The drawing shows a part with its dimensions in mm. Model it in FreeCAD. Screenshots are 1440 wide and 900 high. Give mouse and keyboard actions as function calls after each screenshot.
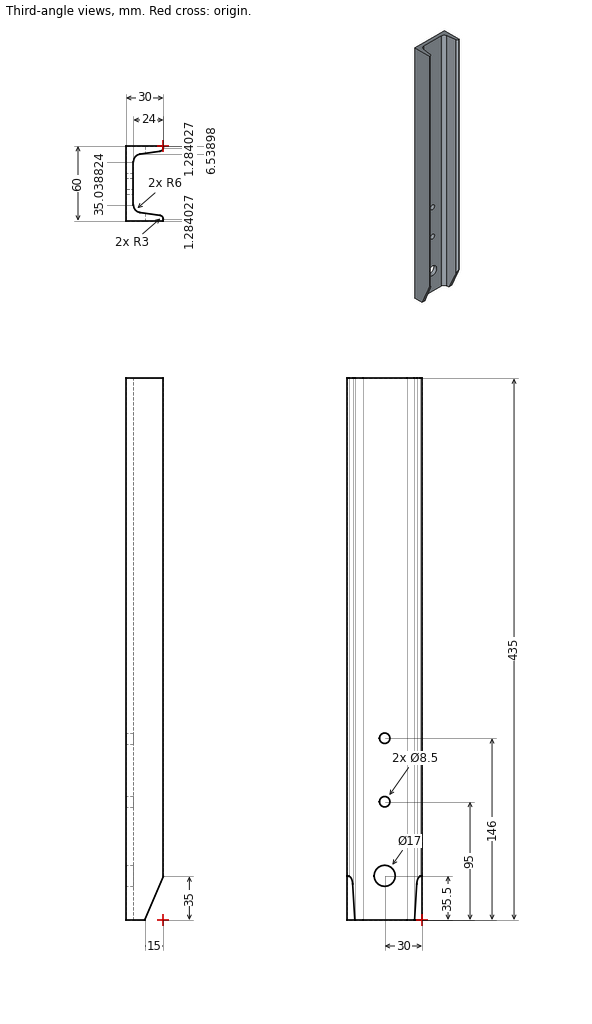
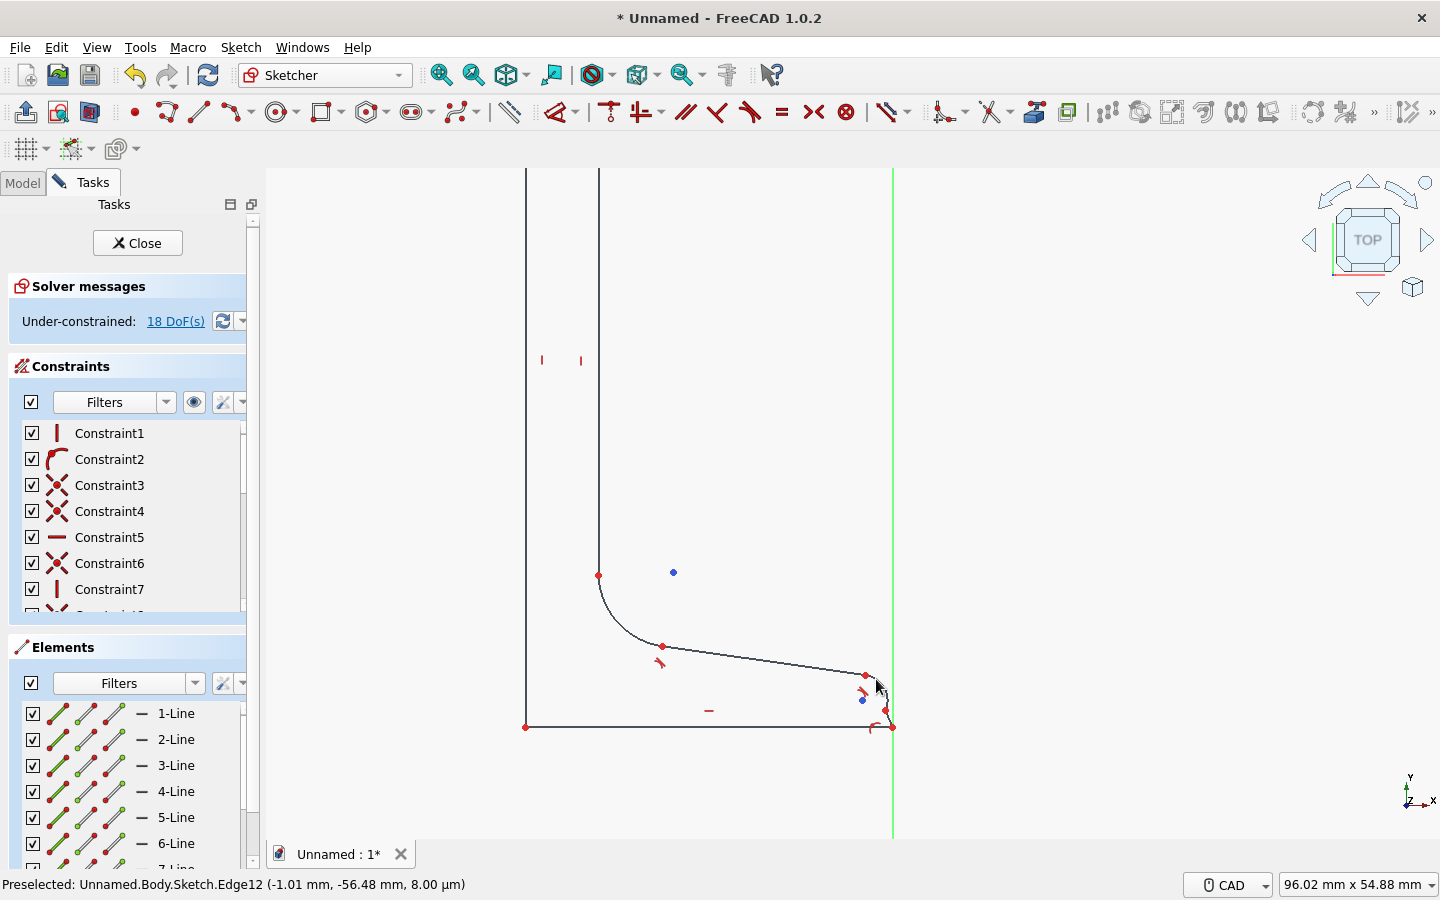
click(599, 446)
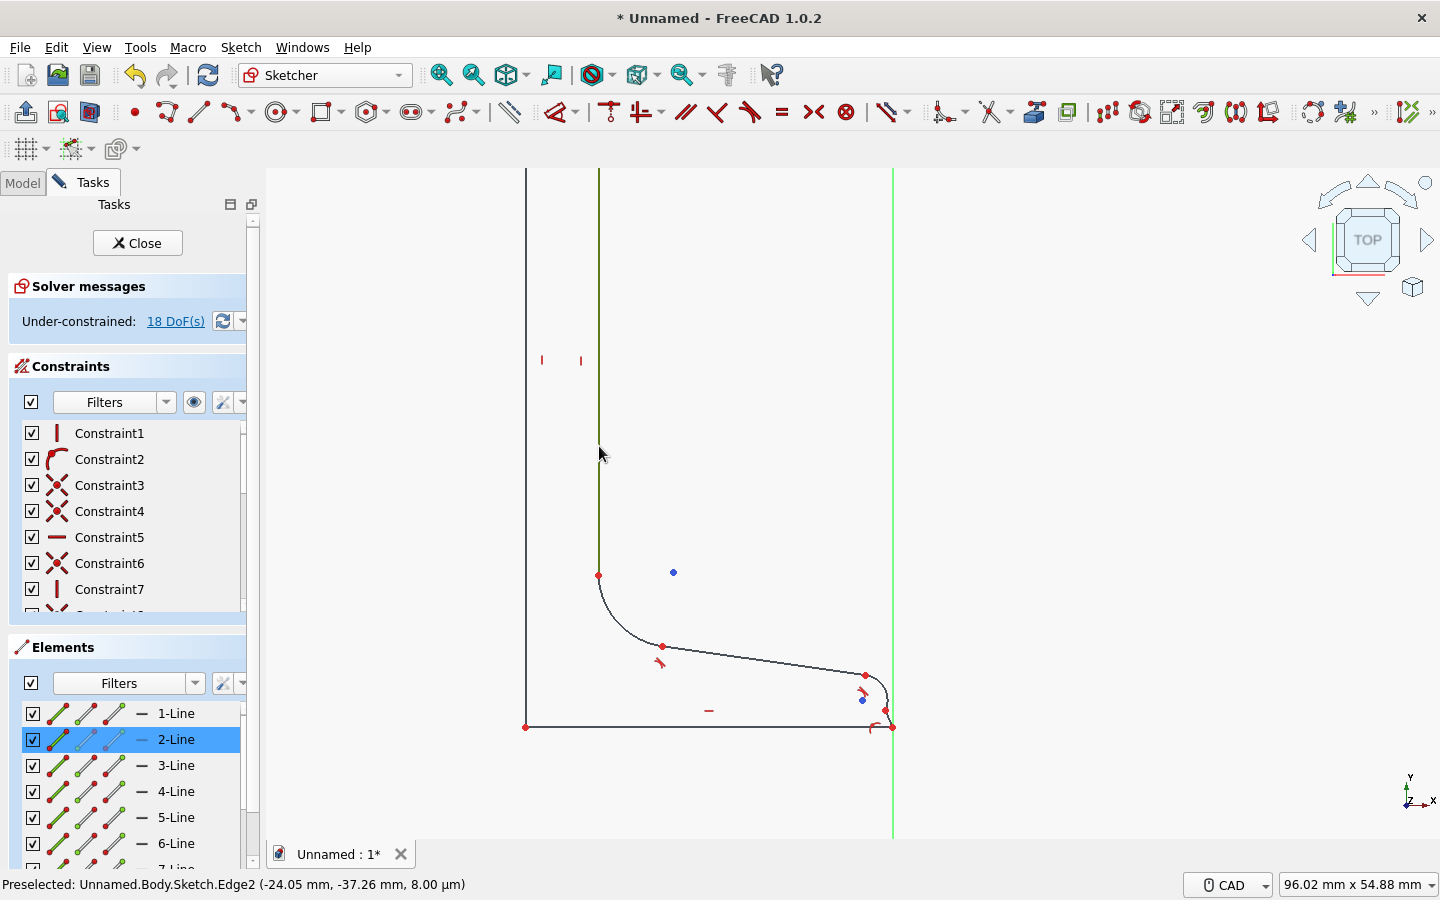
click(606, 605)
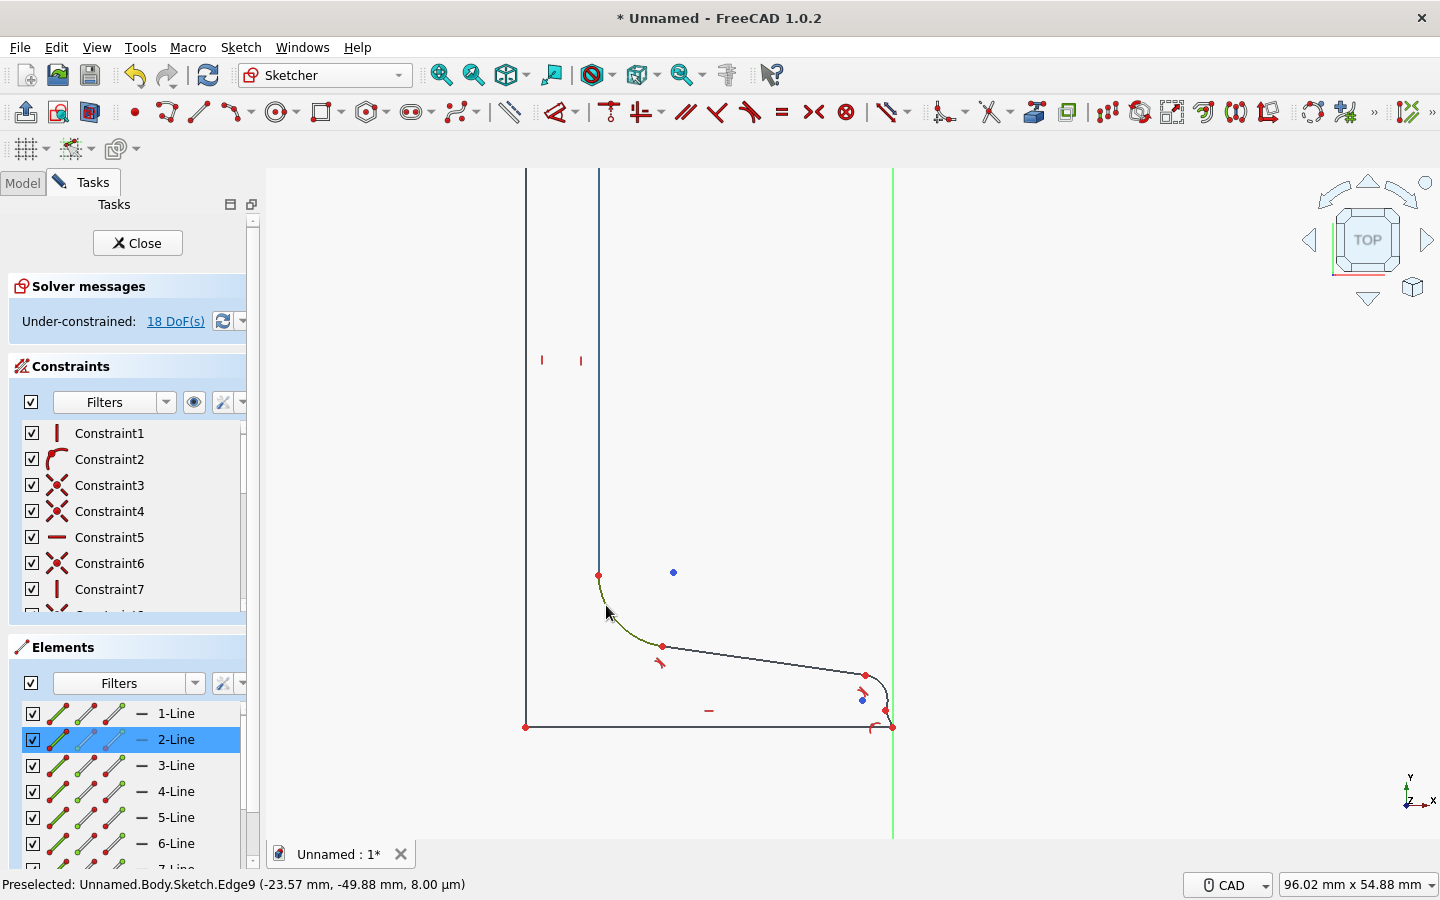
key(t)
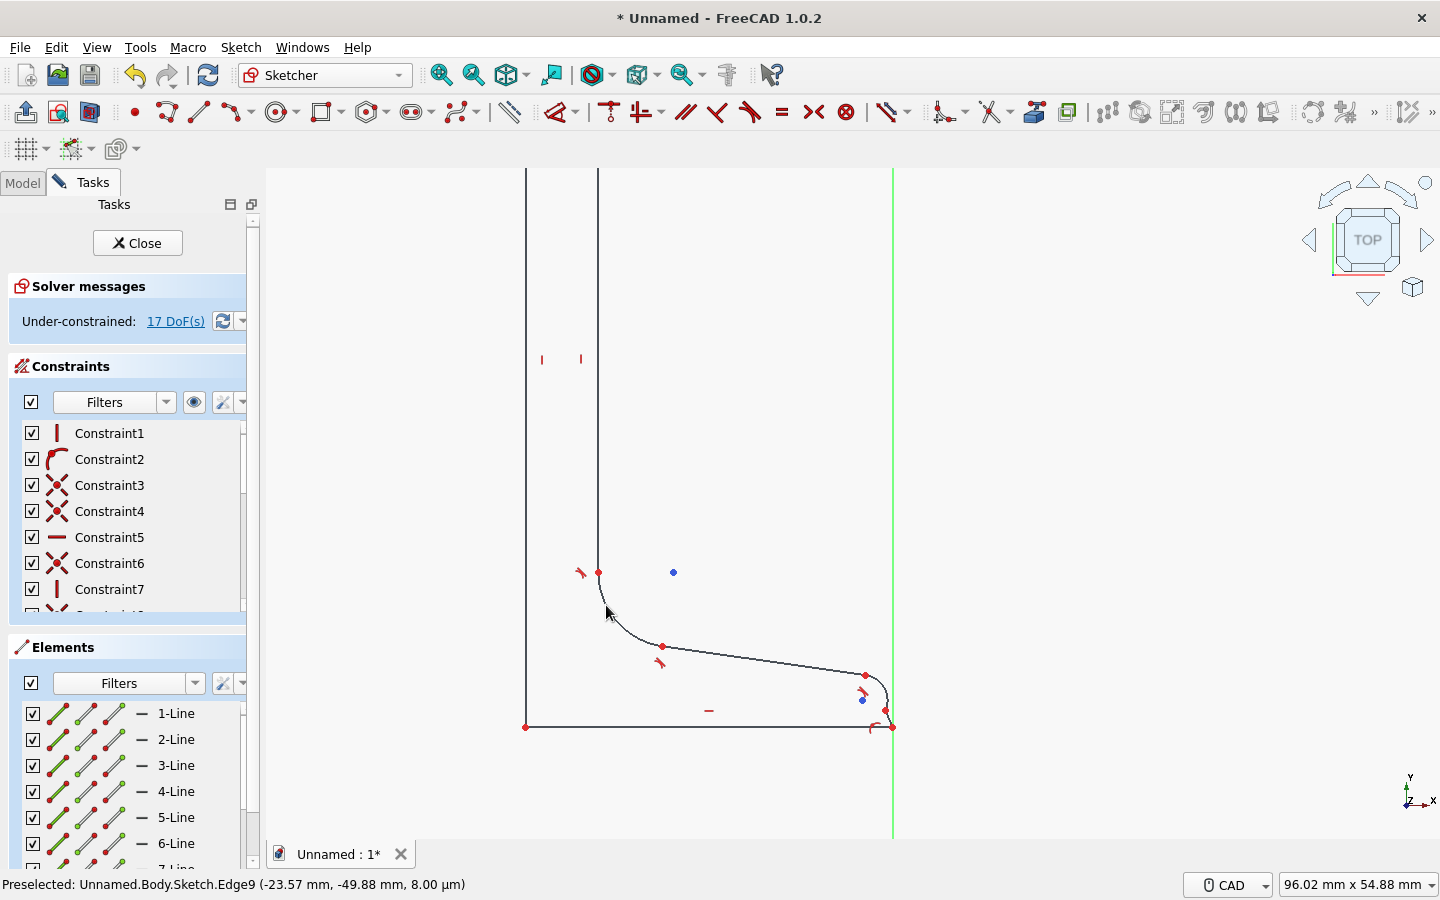
click(598, 444)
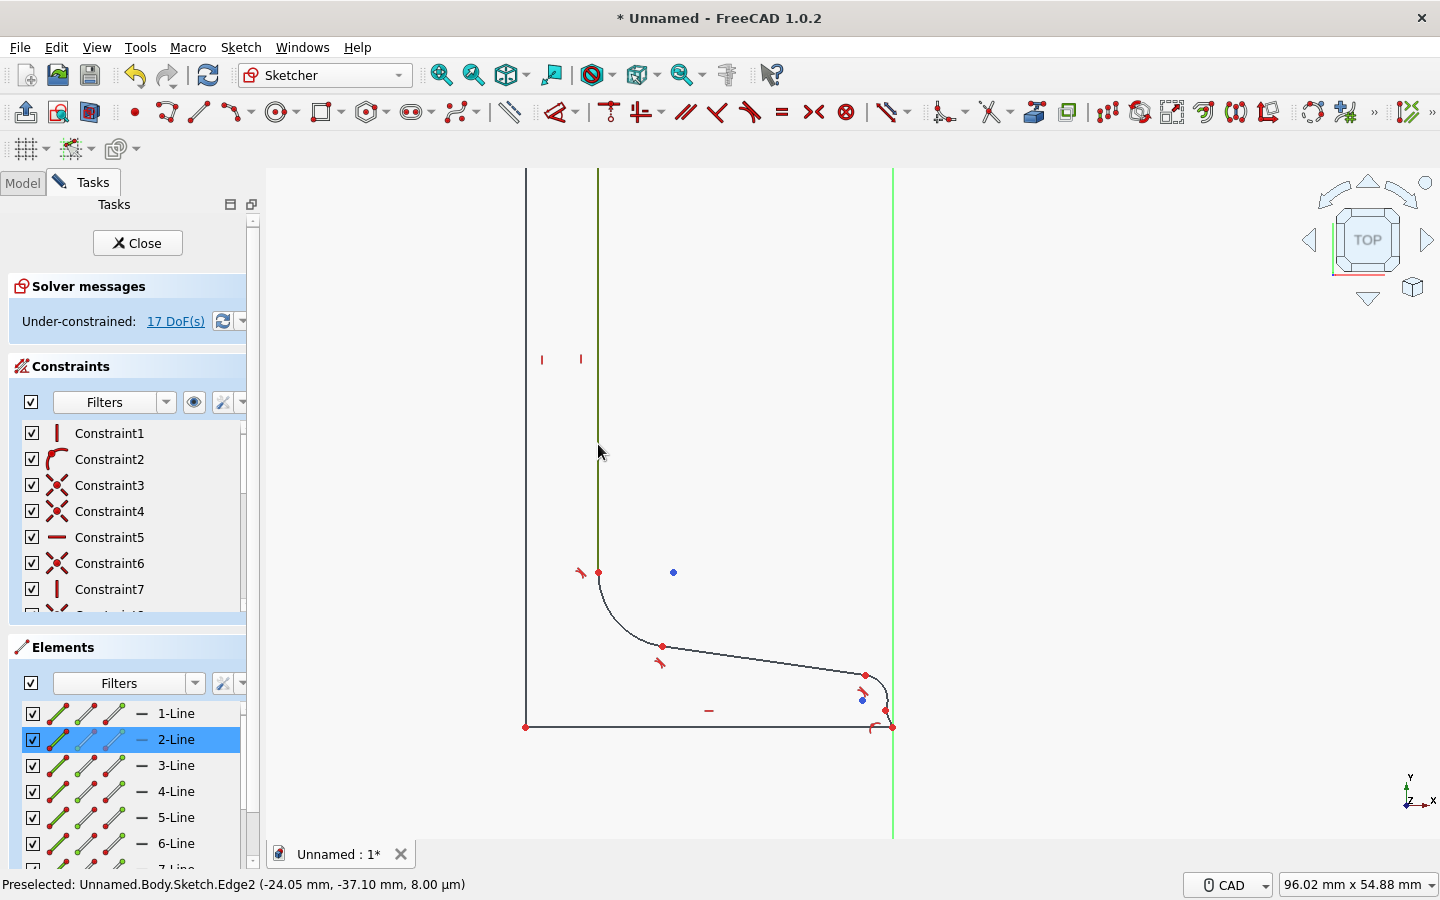
scroll(876, 680, down, 3)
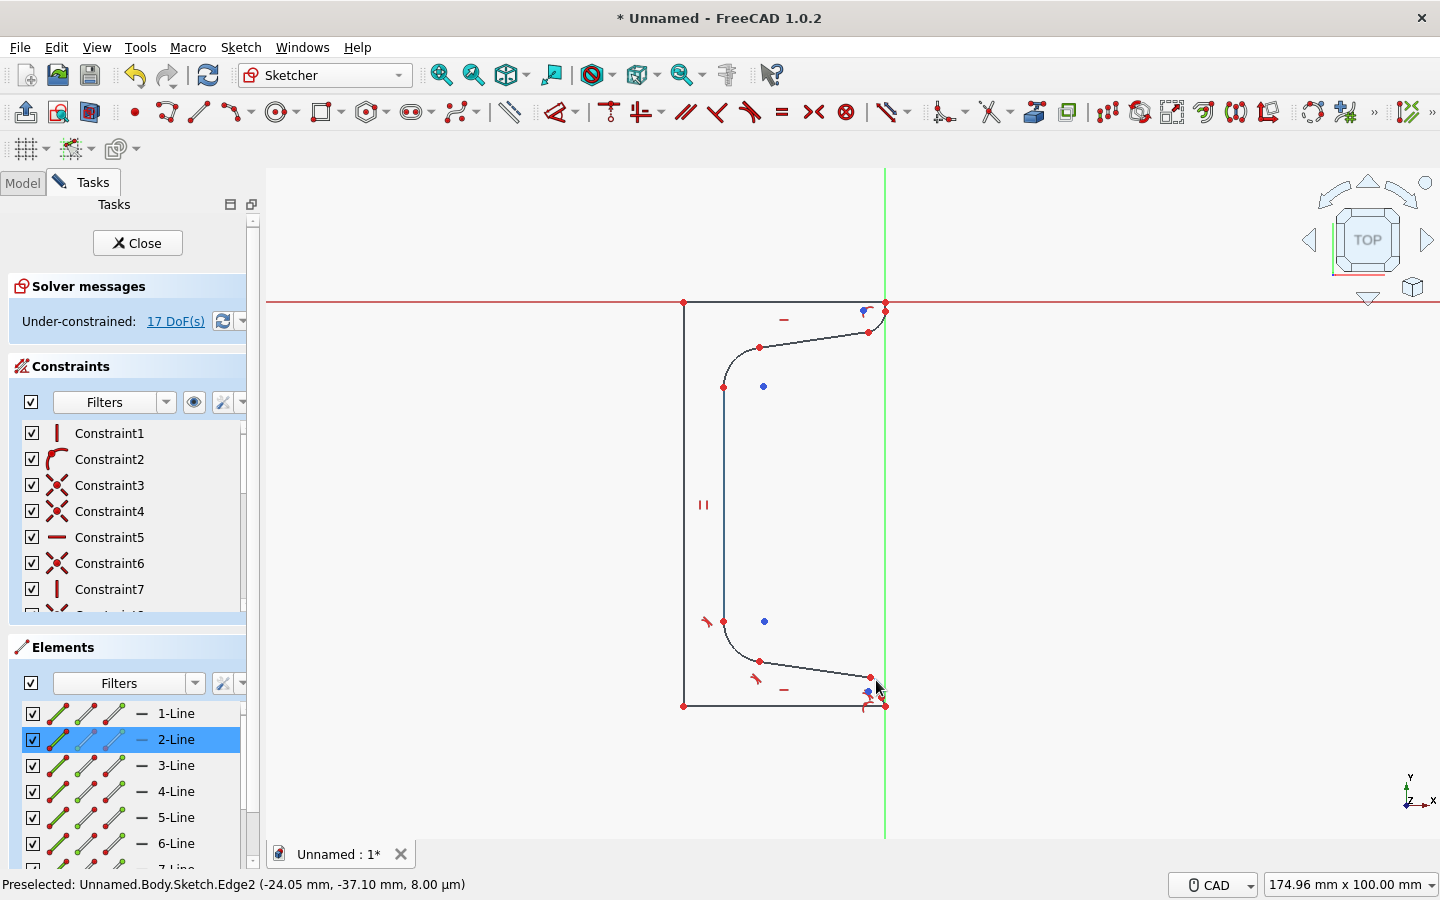
click(743, 353)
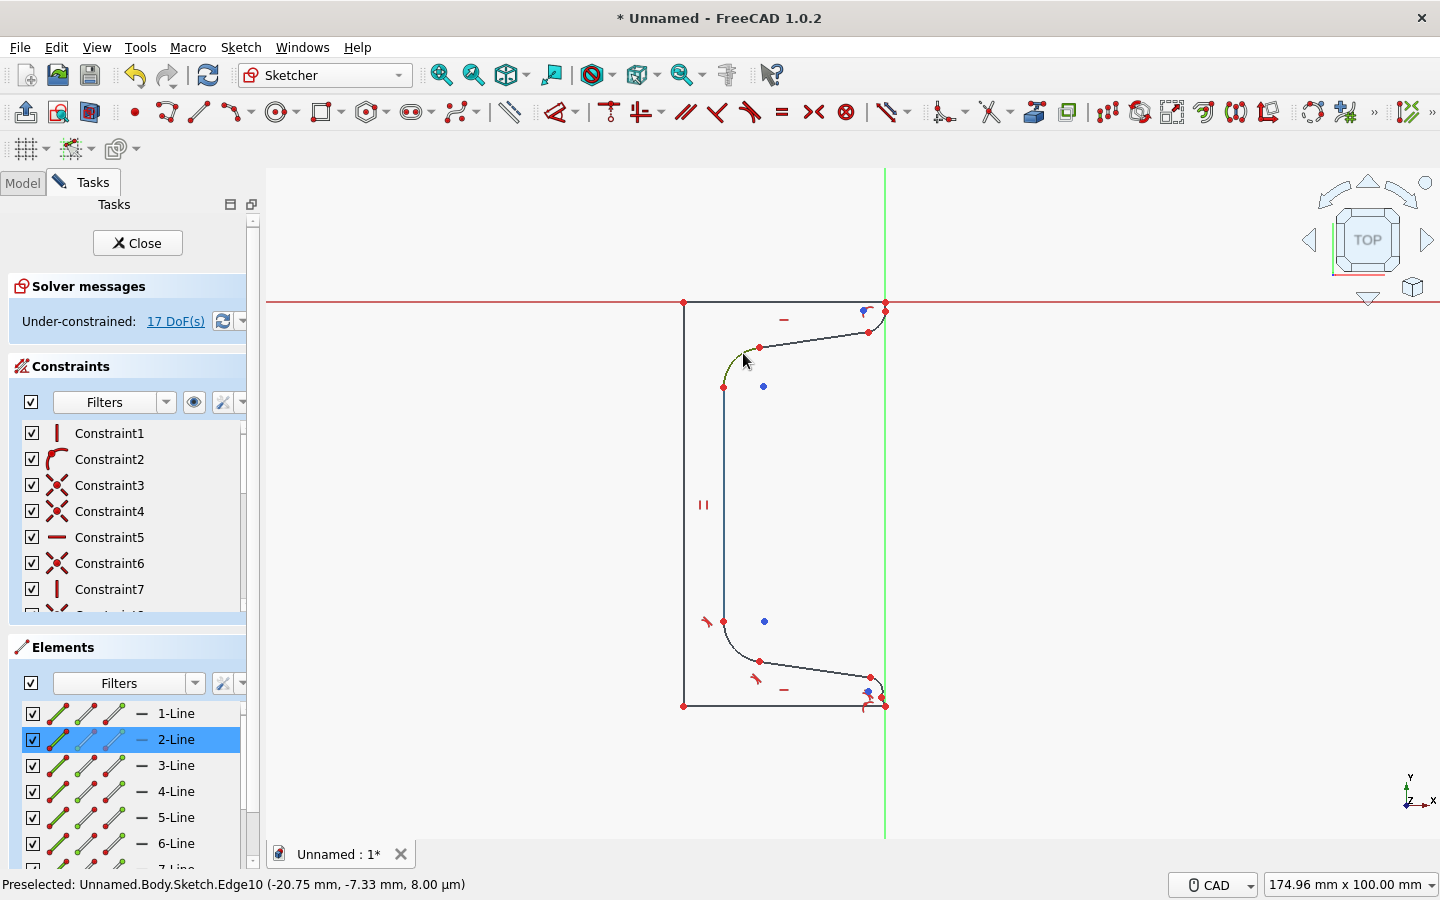
click(750, 112)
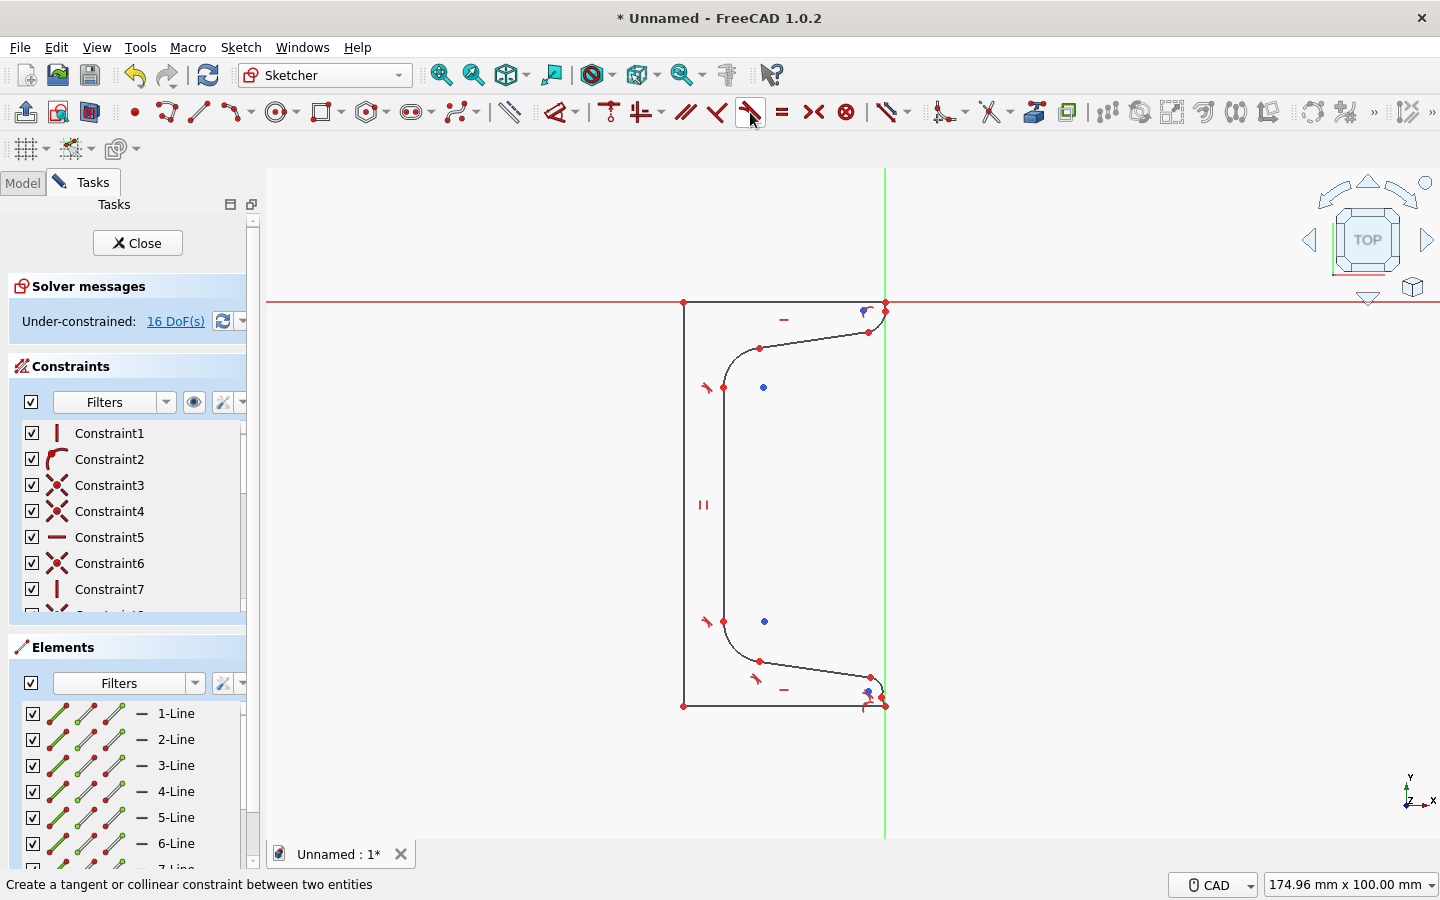
click(792, 343)